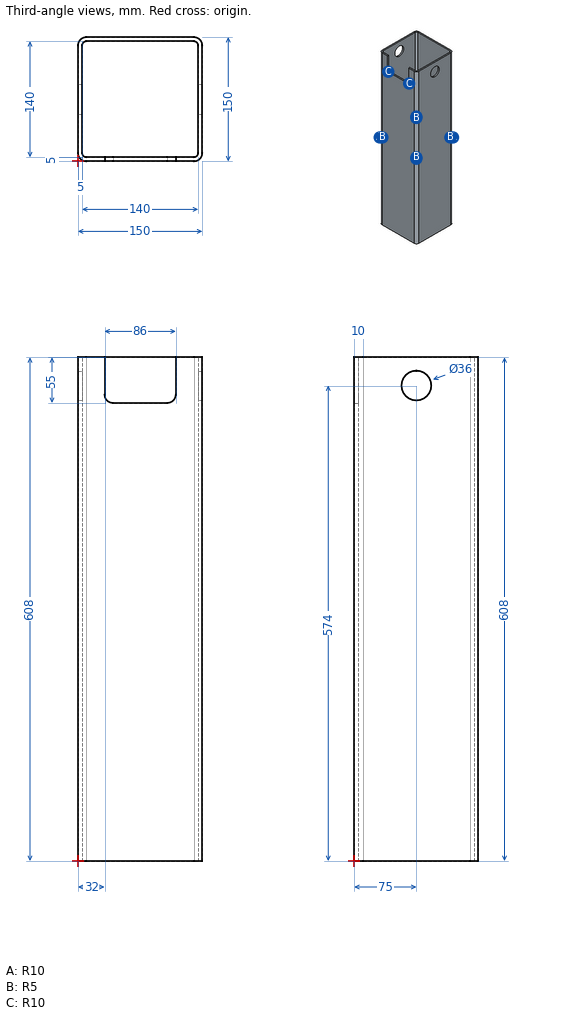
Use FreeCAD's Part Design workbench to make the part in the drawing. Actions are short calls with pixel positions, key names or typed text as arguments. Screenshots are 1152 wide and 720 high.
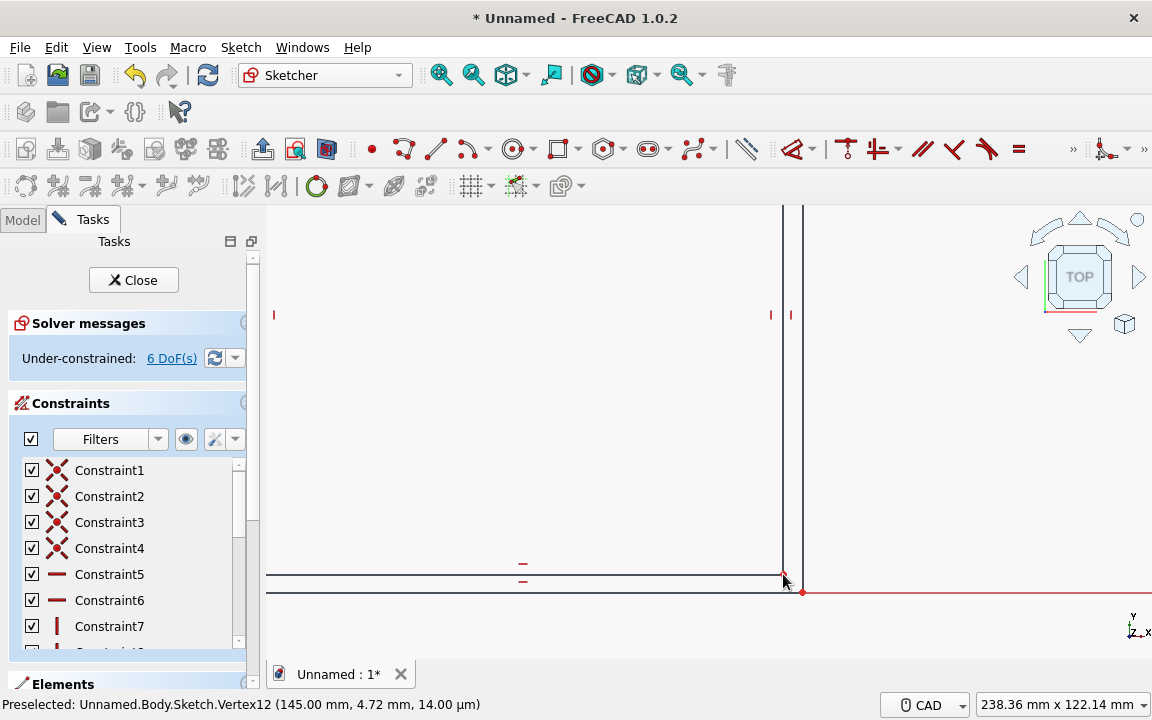
scroll(784, 576, down, 3)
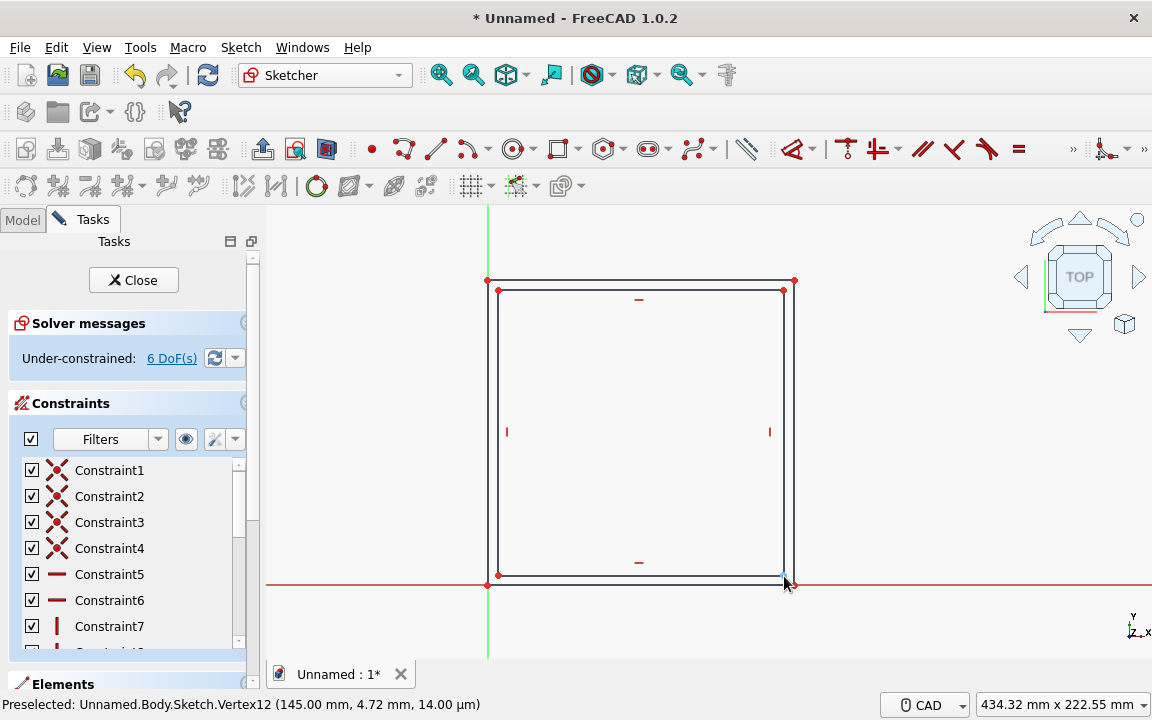
scroll(498, 290, up, 7)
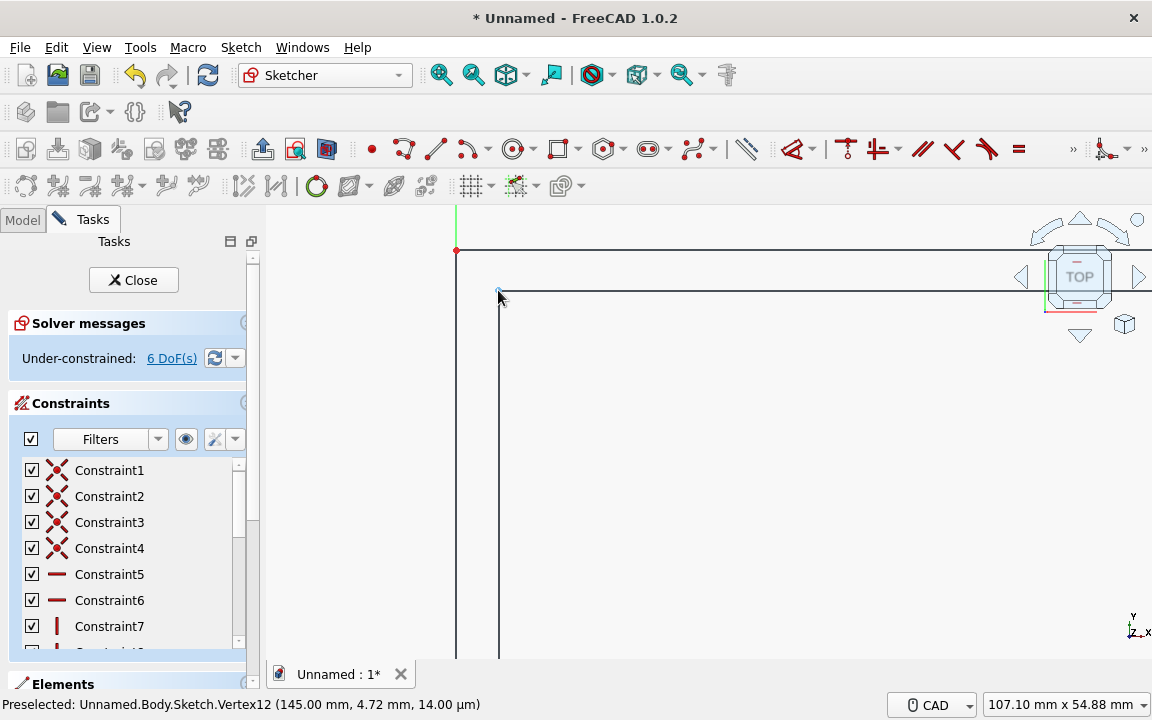
click(499, 291)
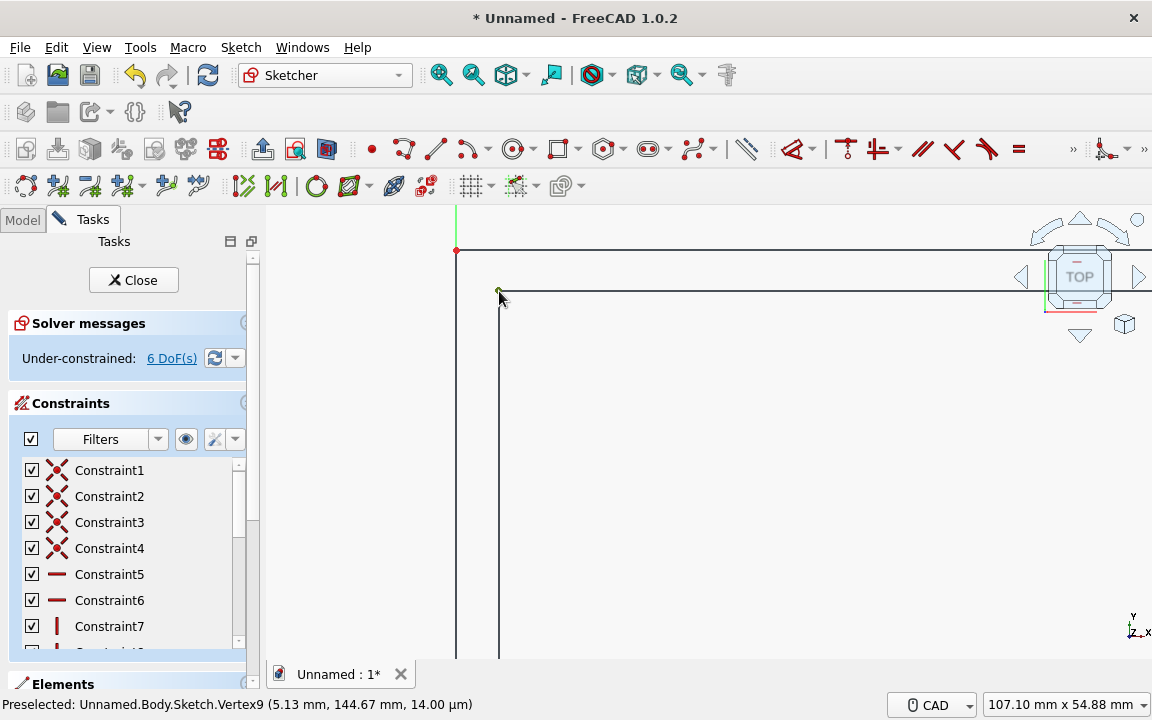
key(l)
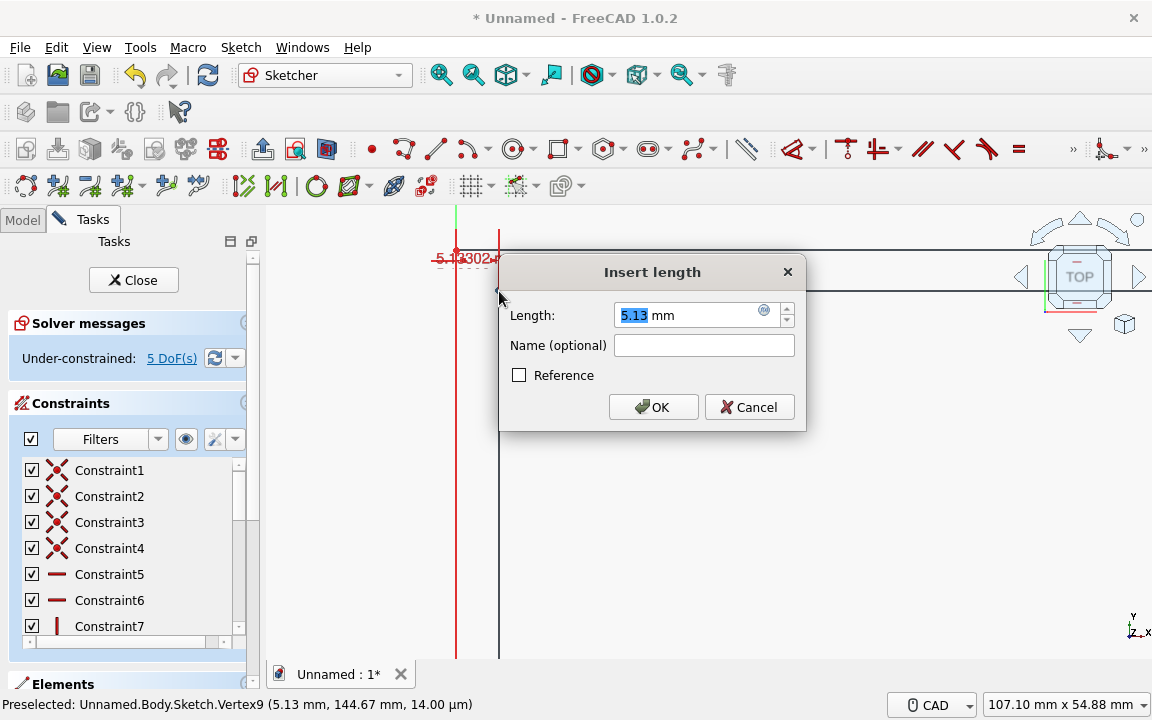
text(5)
key(Return)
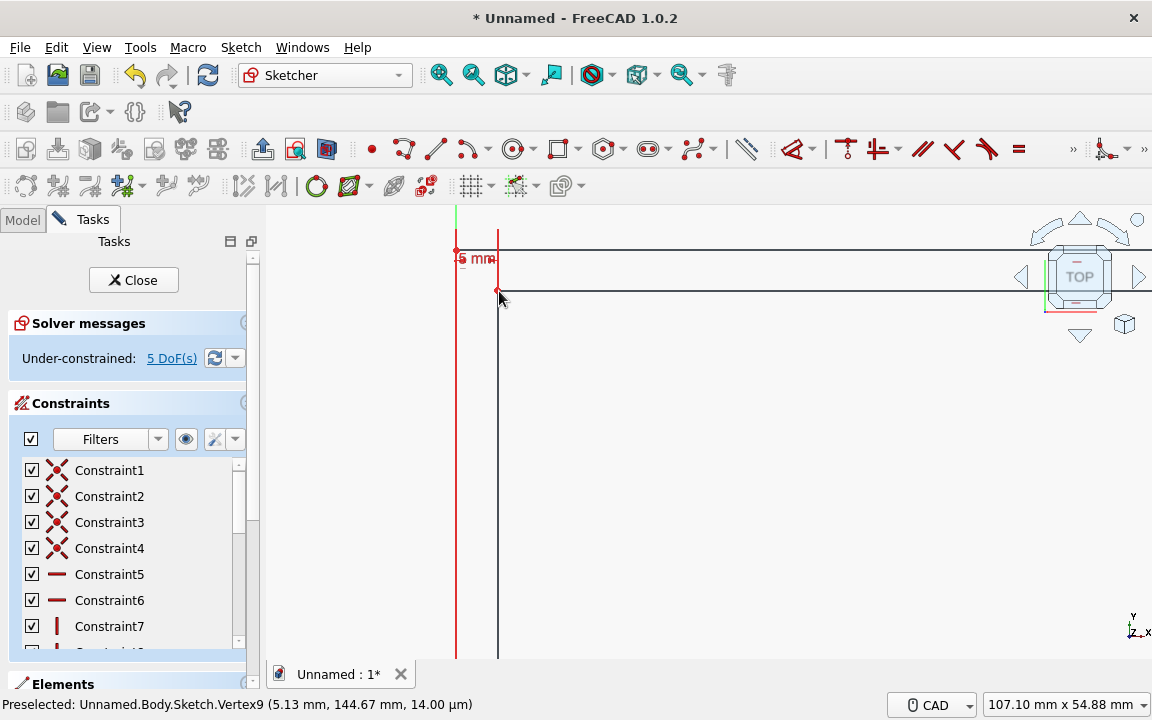
scroll(498, 290, down, 7)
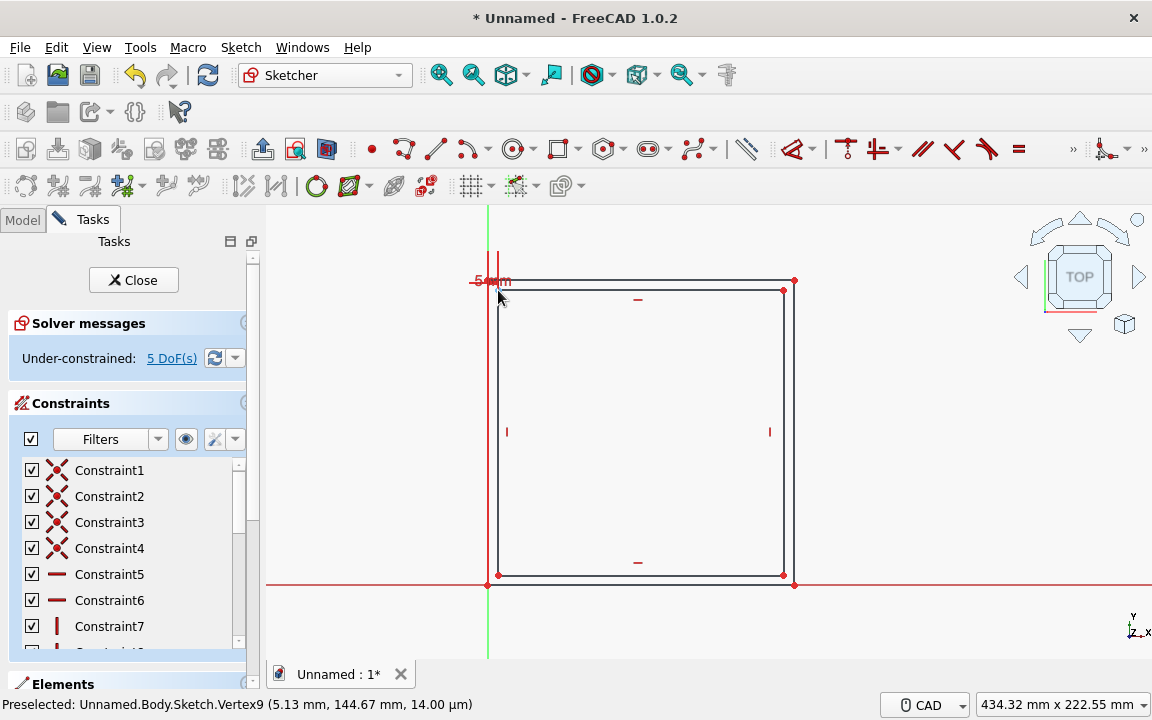
scroll(498, 576, up, 7)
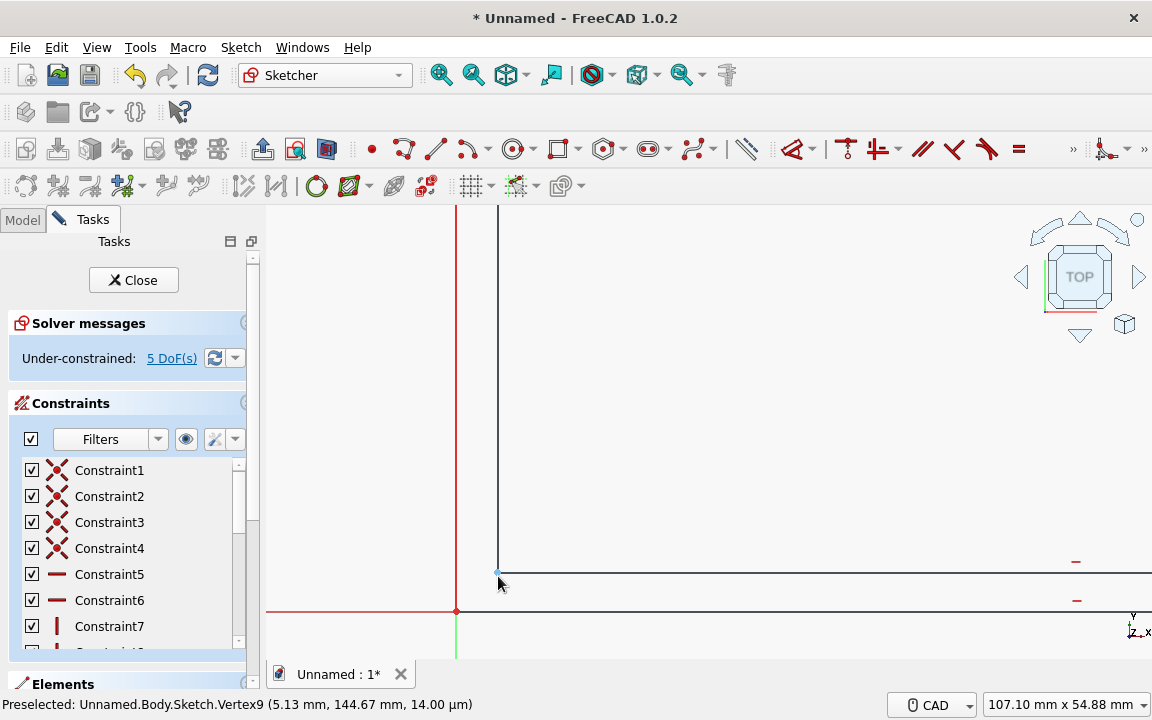
click(498, 573)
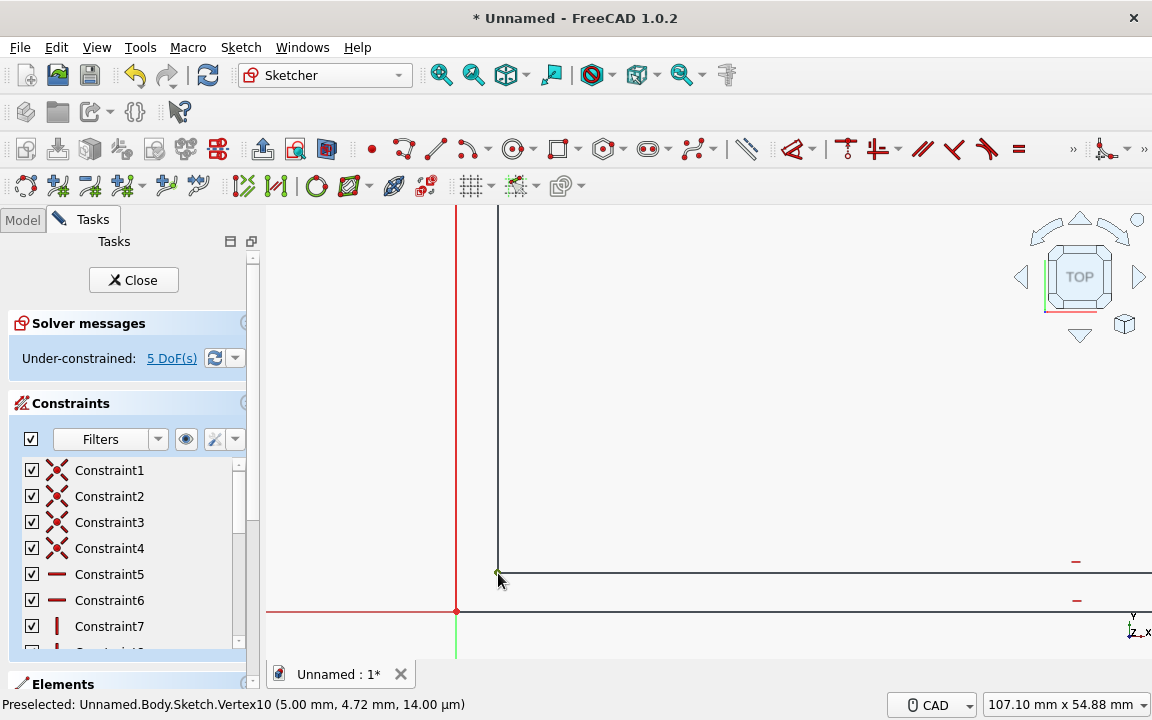
click(814, 150)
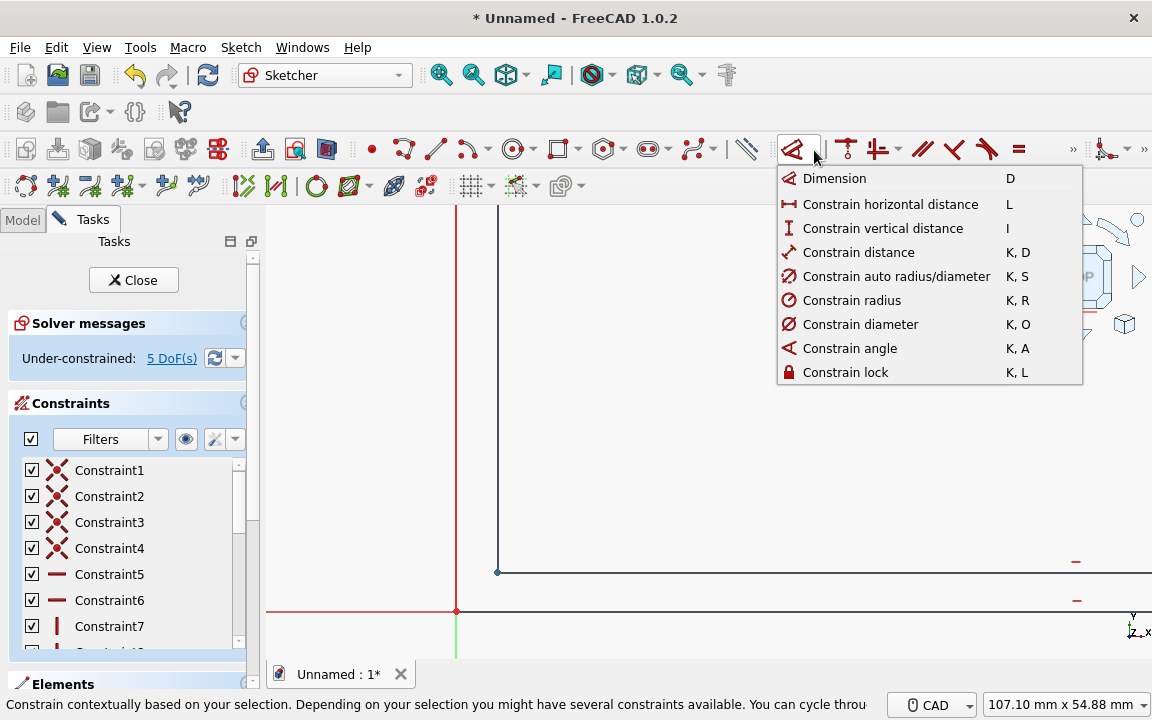
click(930, 228)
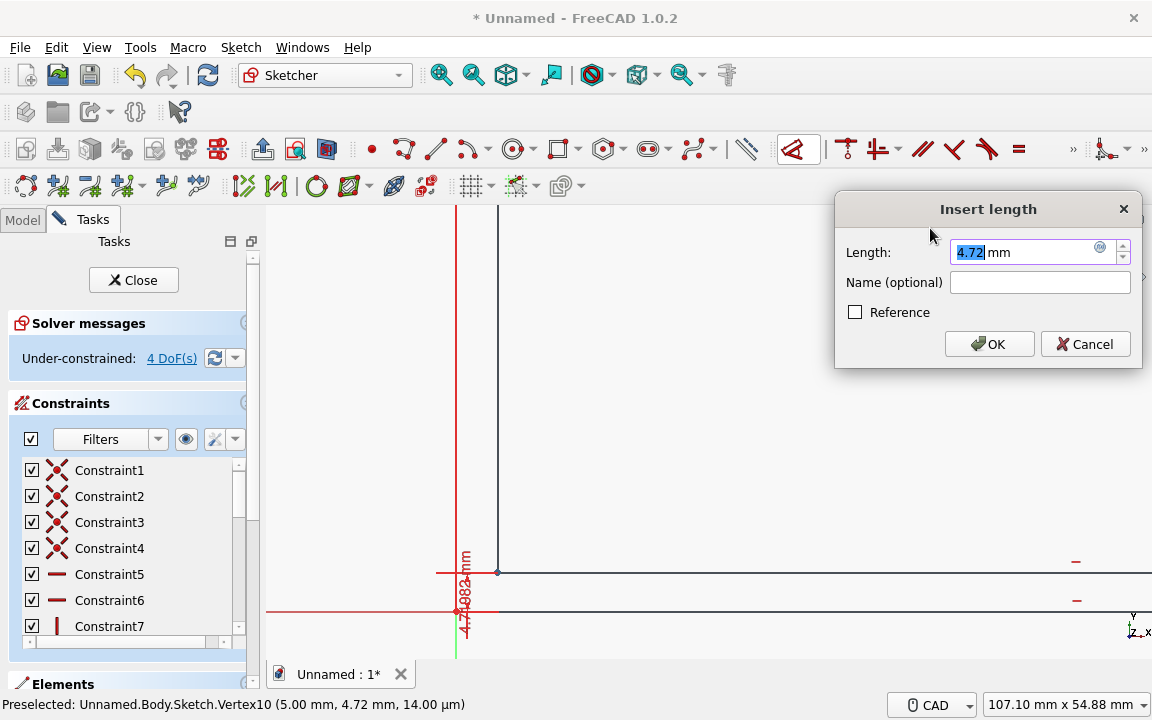
text(5)
key(Return)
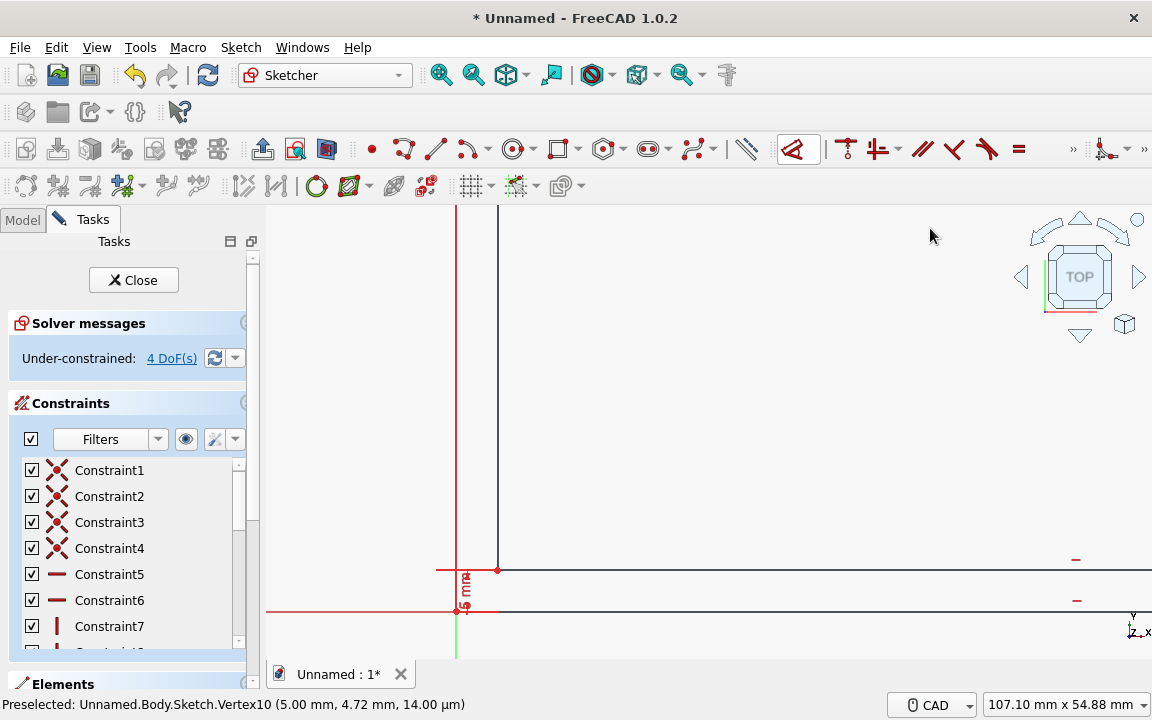
scroll(498, 576, down, 7)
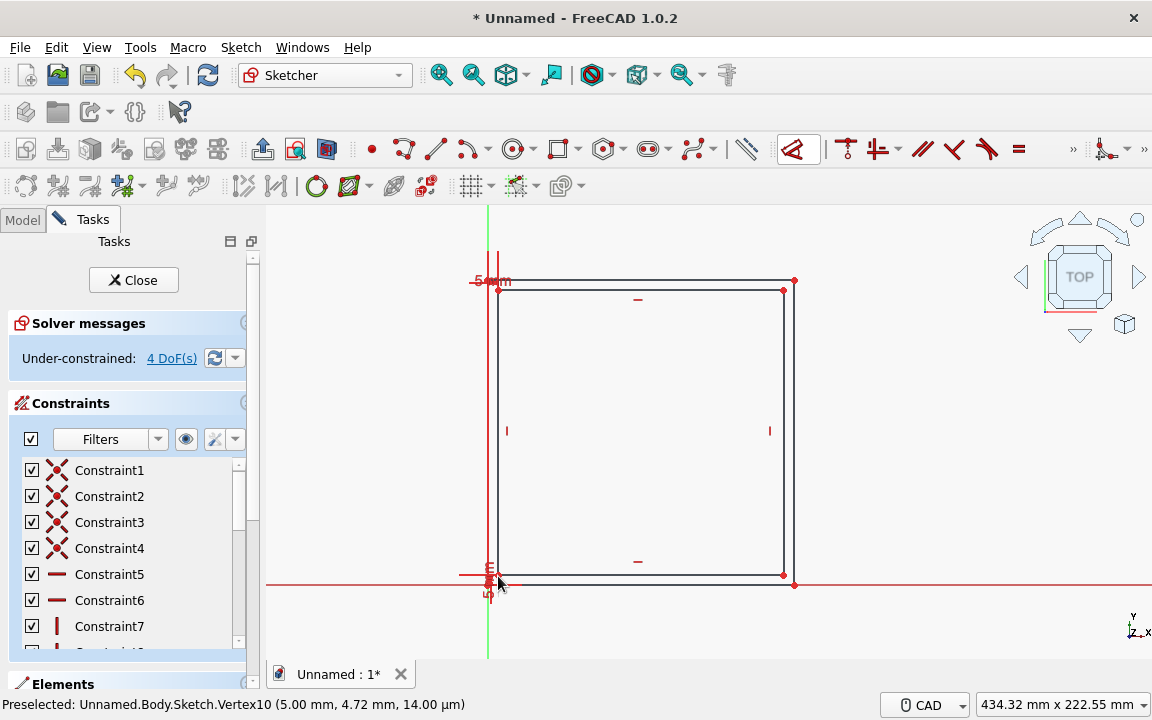
scroll(580, 585, up, 2)